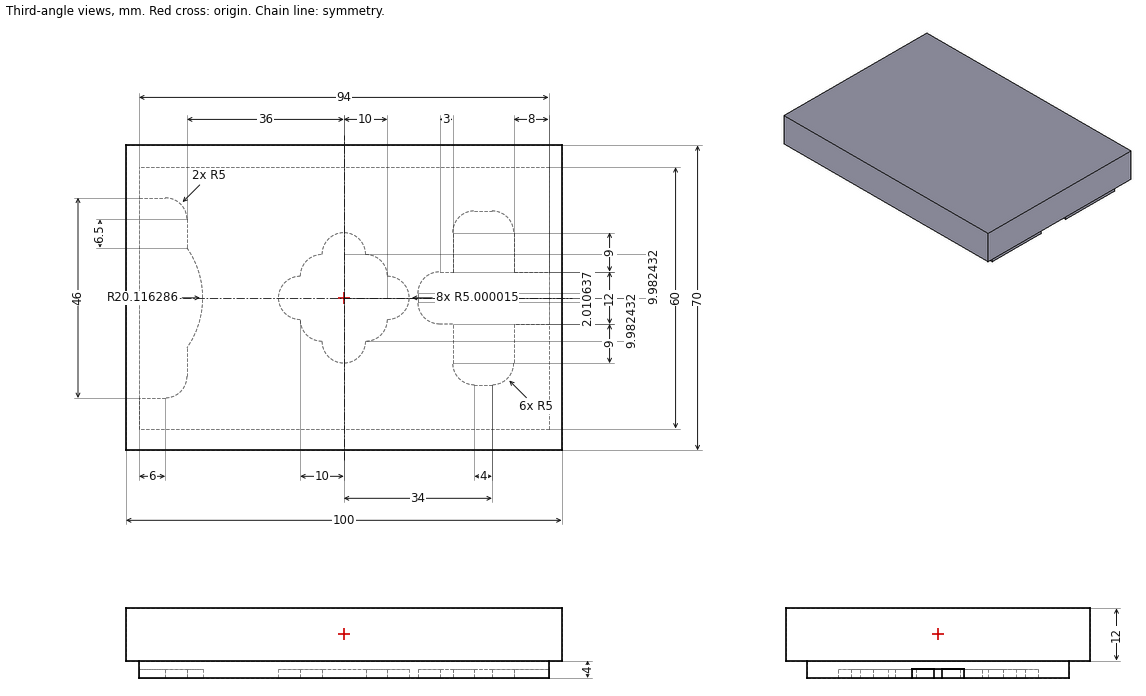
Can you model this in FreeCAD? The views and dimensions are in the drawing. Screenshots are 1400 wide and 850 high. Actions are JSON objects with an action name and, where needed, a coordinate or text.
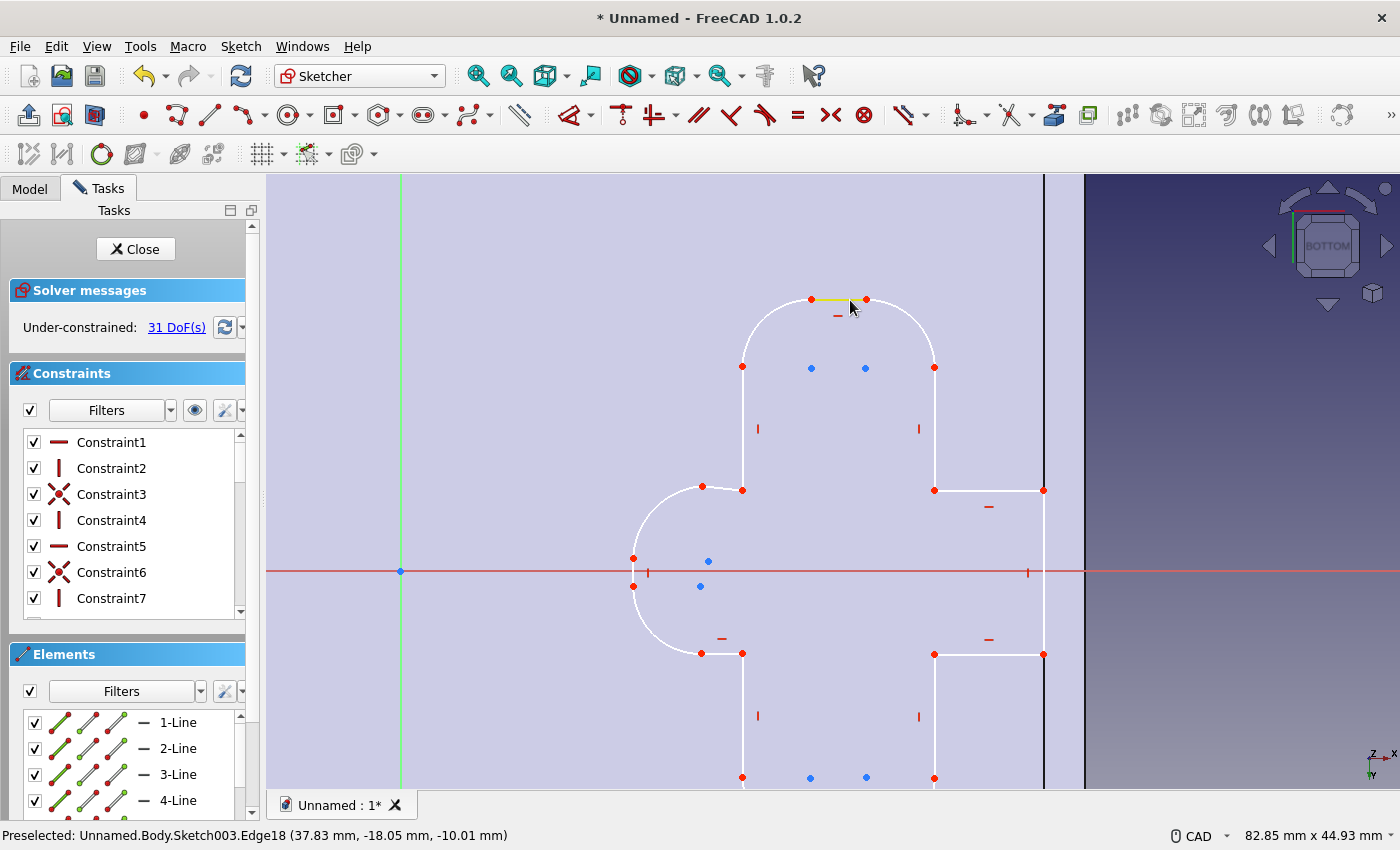
{"action": "left_click", "coordinate": [850, 300]}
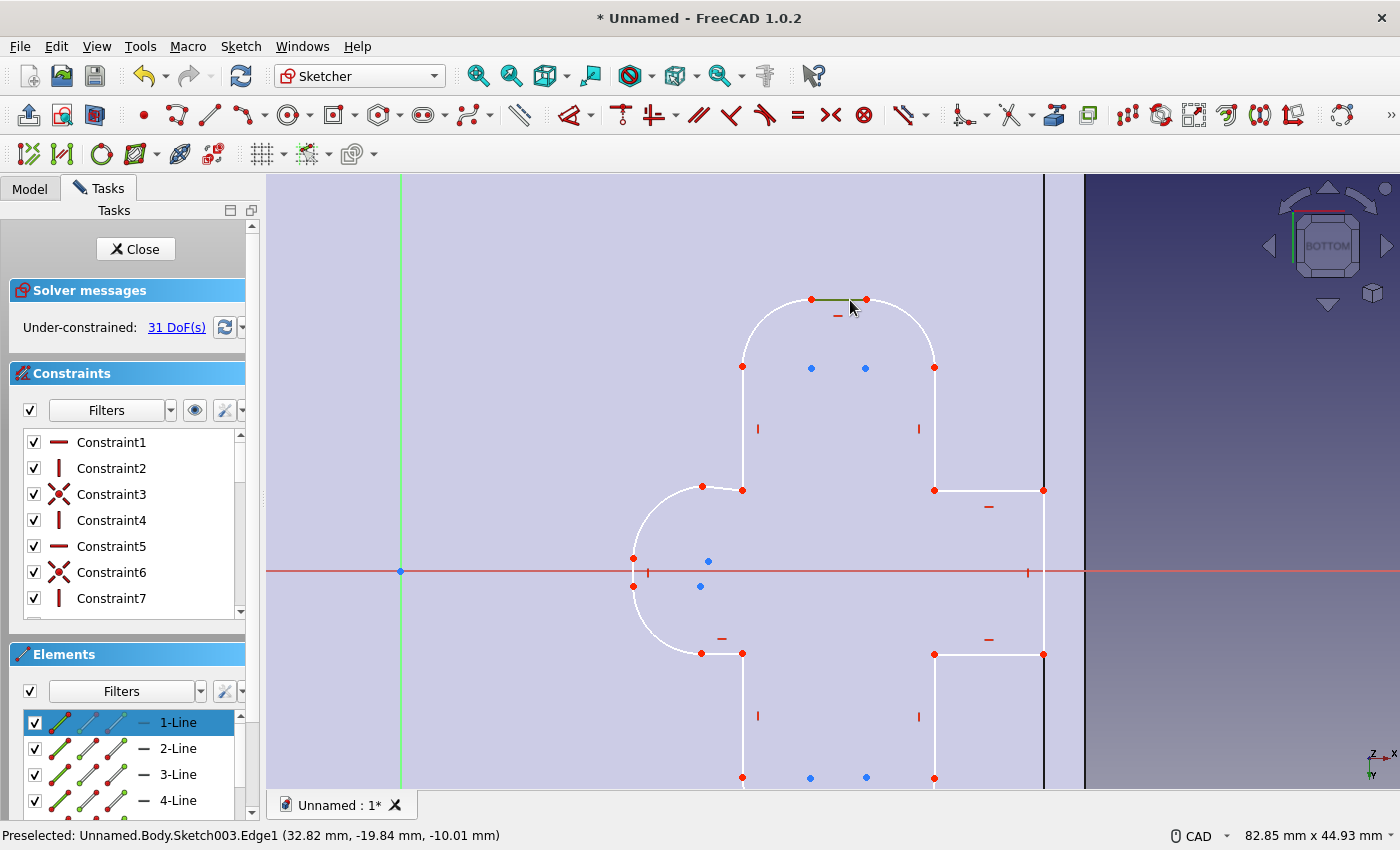
{"action": "left_click", "coordinate": [780, 307]}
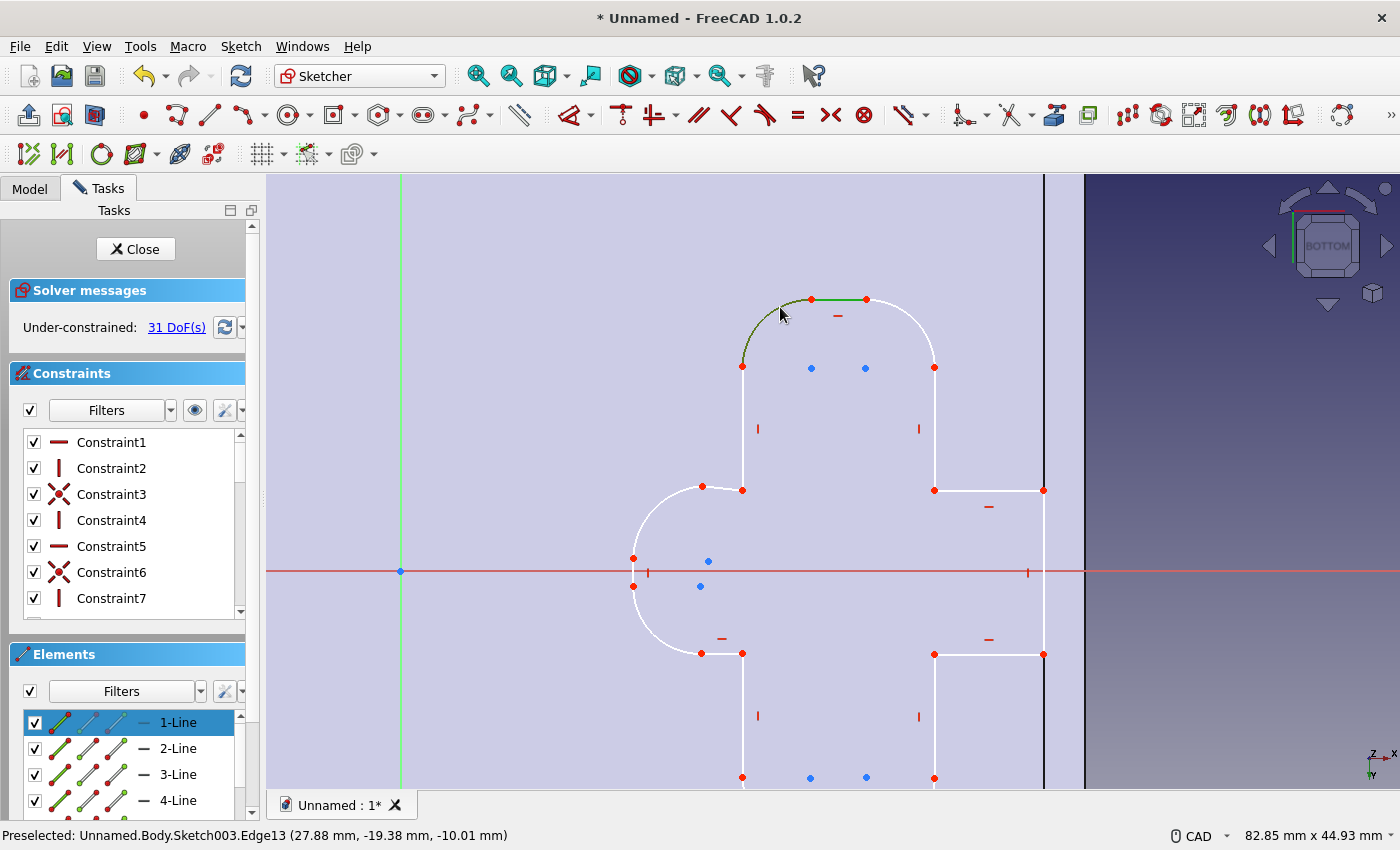
{"action": "left_click", "coordinate": [765, 116]}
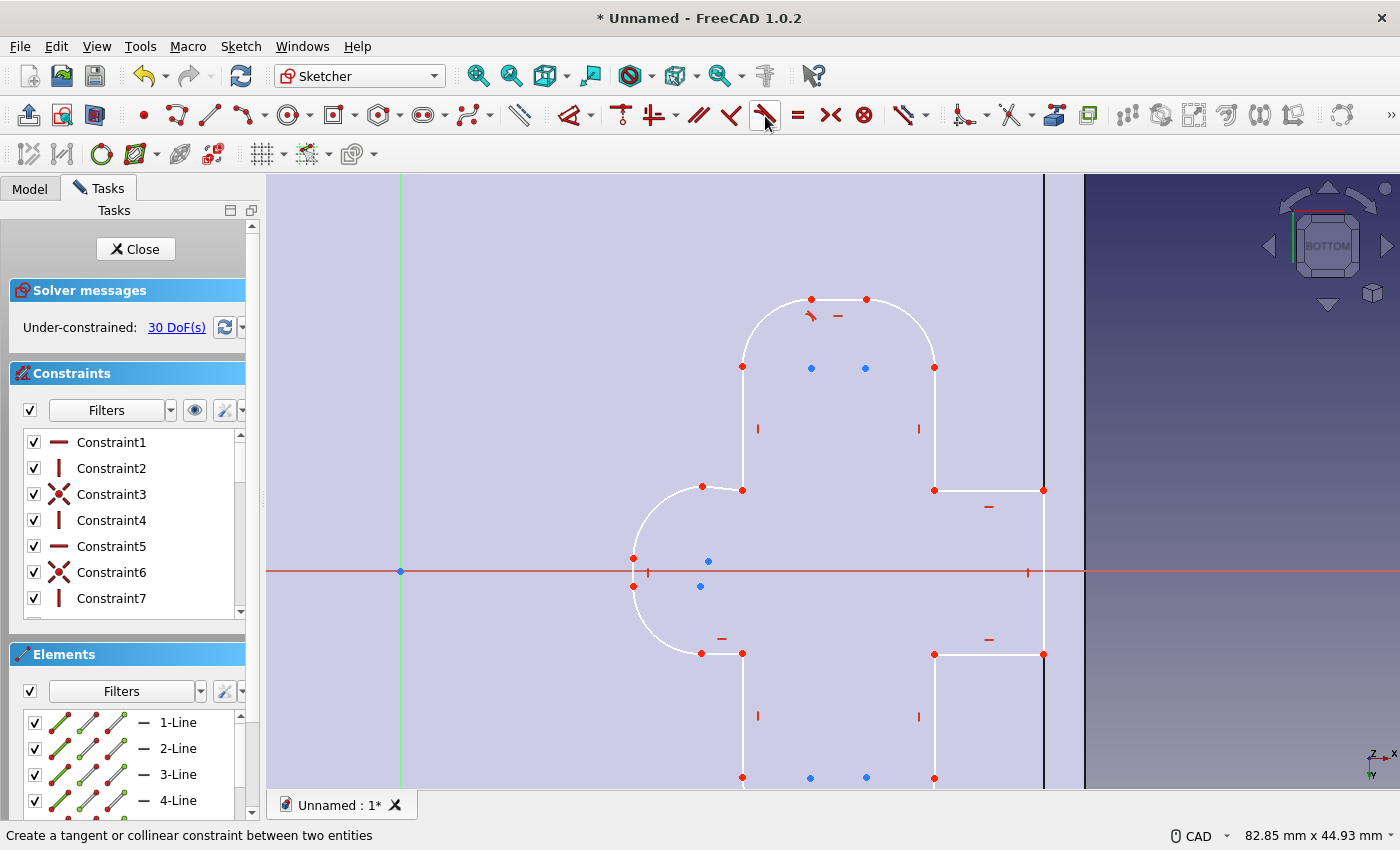
{"action": "left_click", "coordinate": [850, 300]}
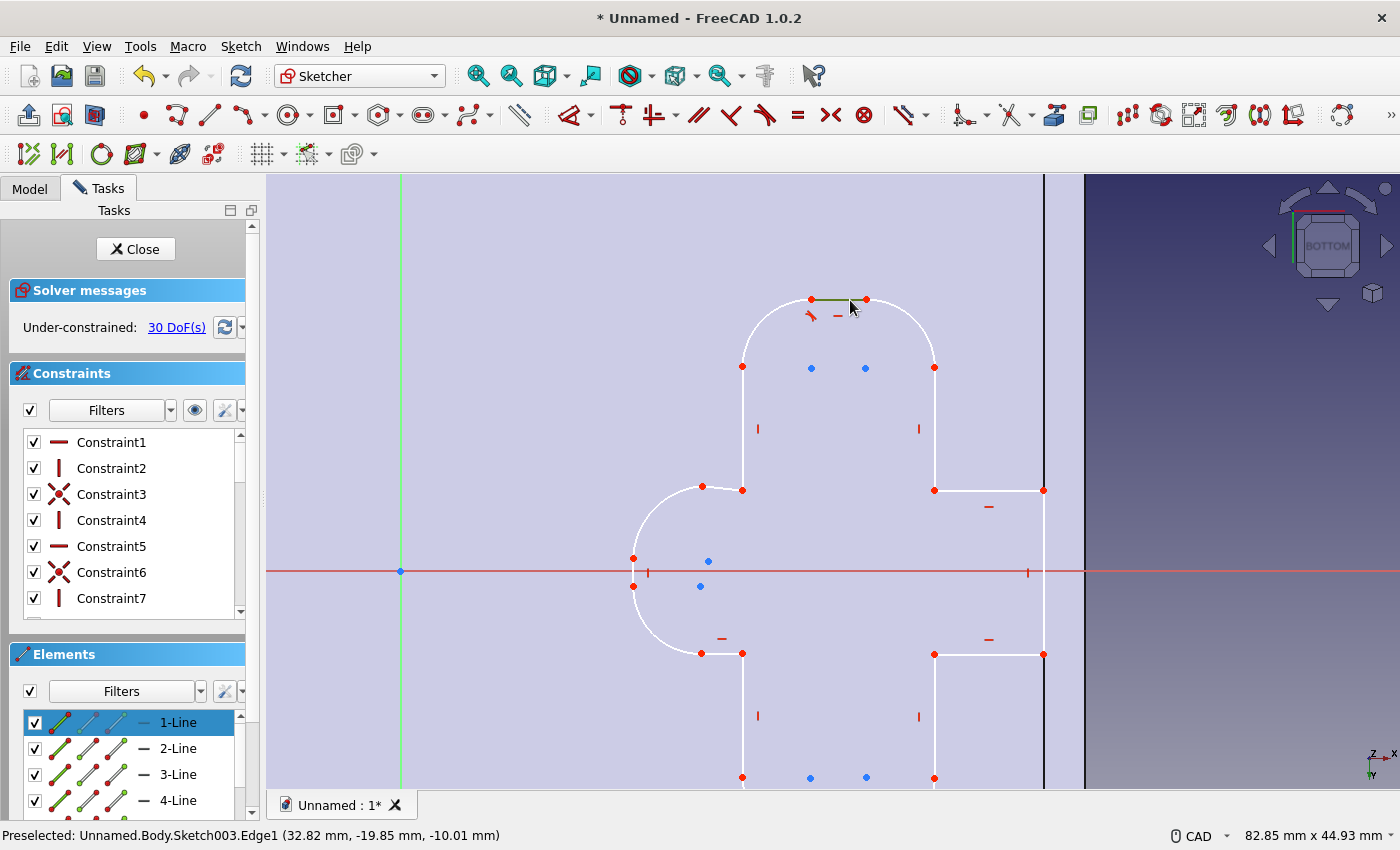
{"action": "left_click", "coordinate": [927, 336]}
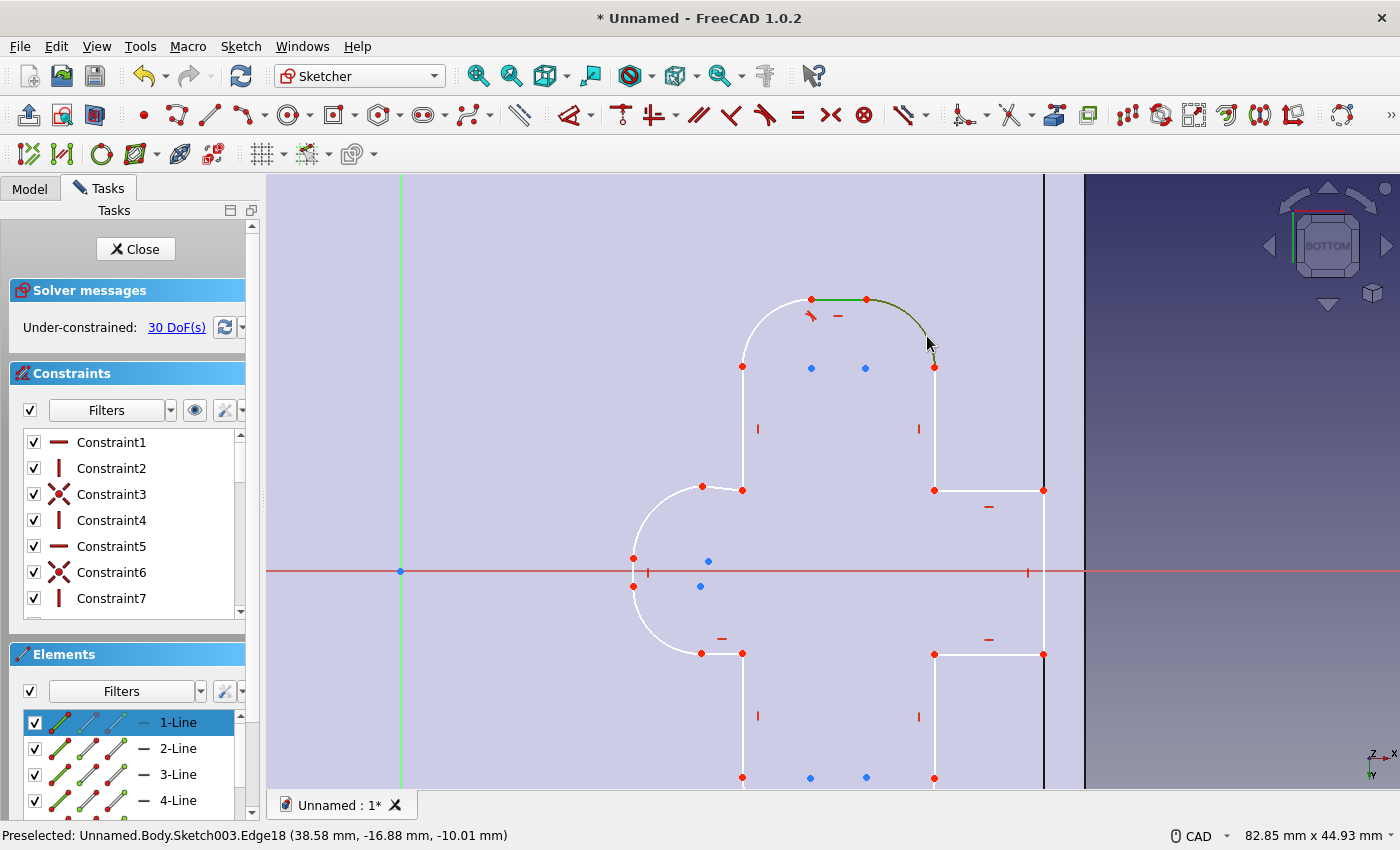
{"action": "left_click", "coordinate": [765, 116]}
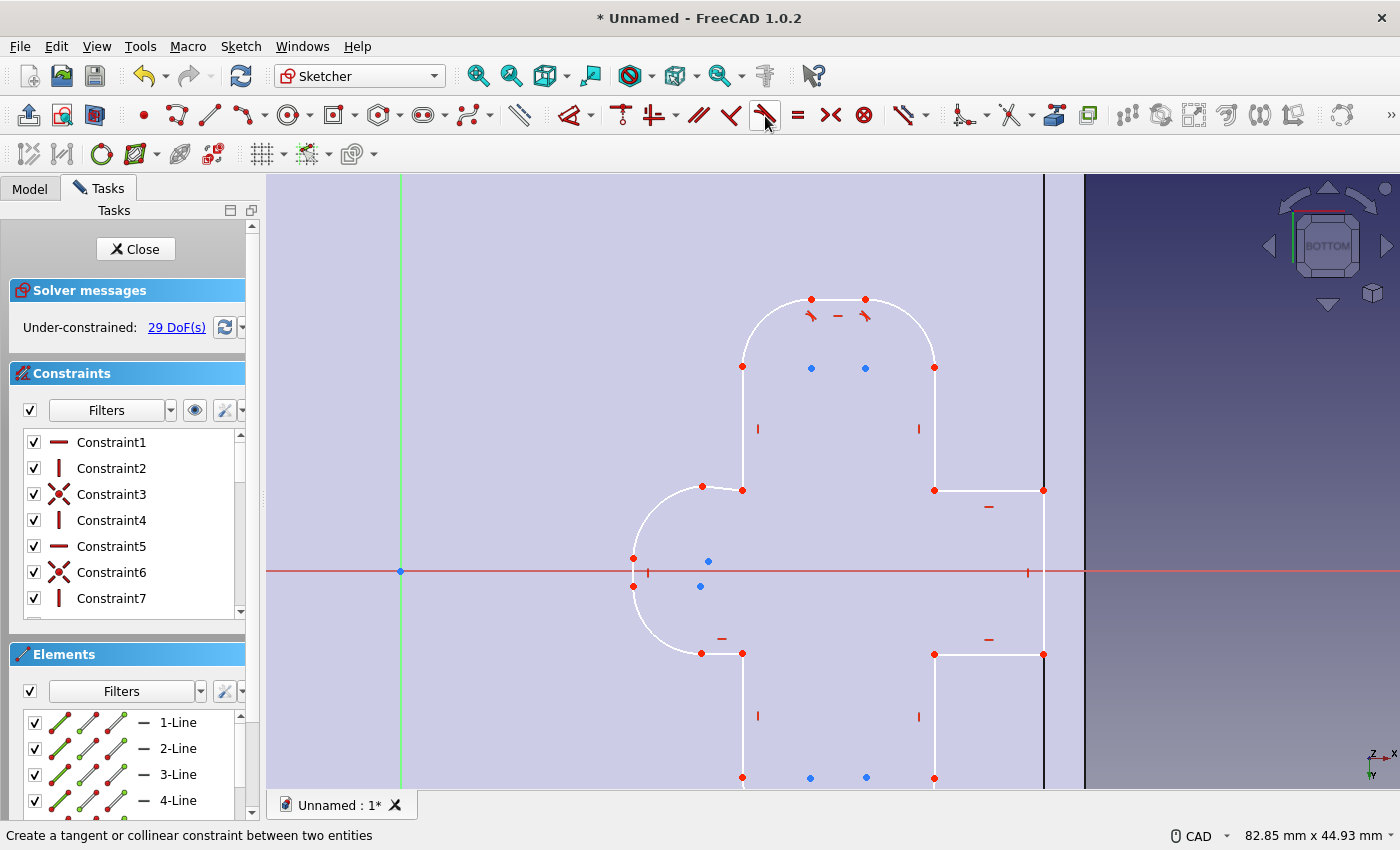
{"action": "left_click", "coordinate": [743, 404]}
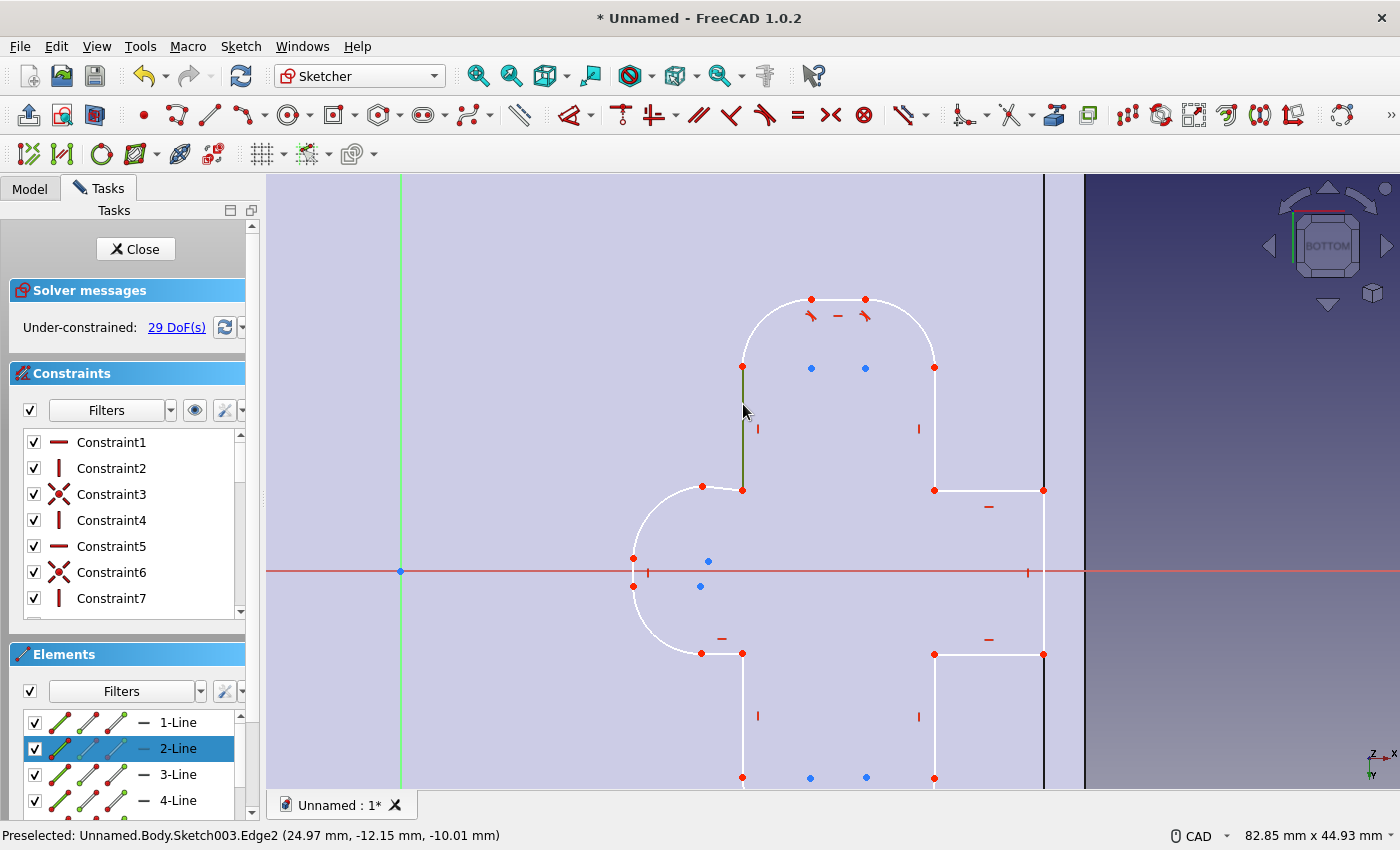
{"action": "left_click", "coordinate": [780, 307]}